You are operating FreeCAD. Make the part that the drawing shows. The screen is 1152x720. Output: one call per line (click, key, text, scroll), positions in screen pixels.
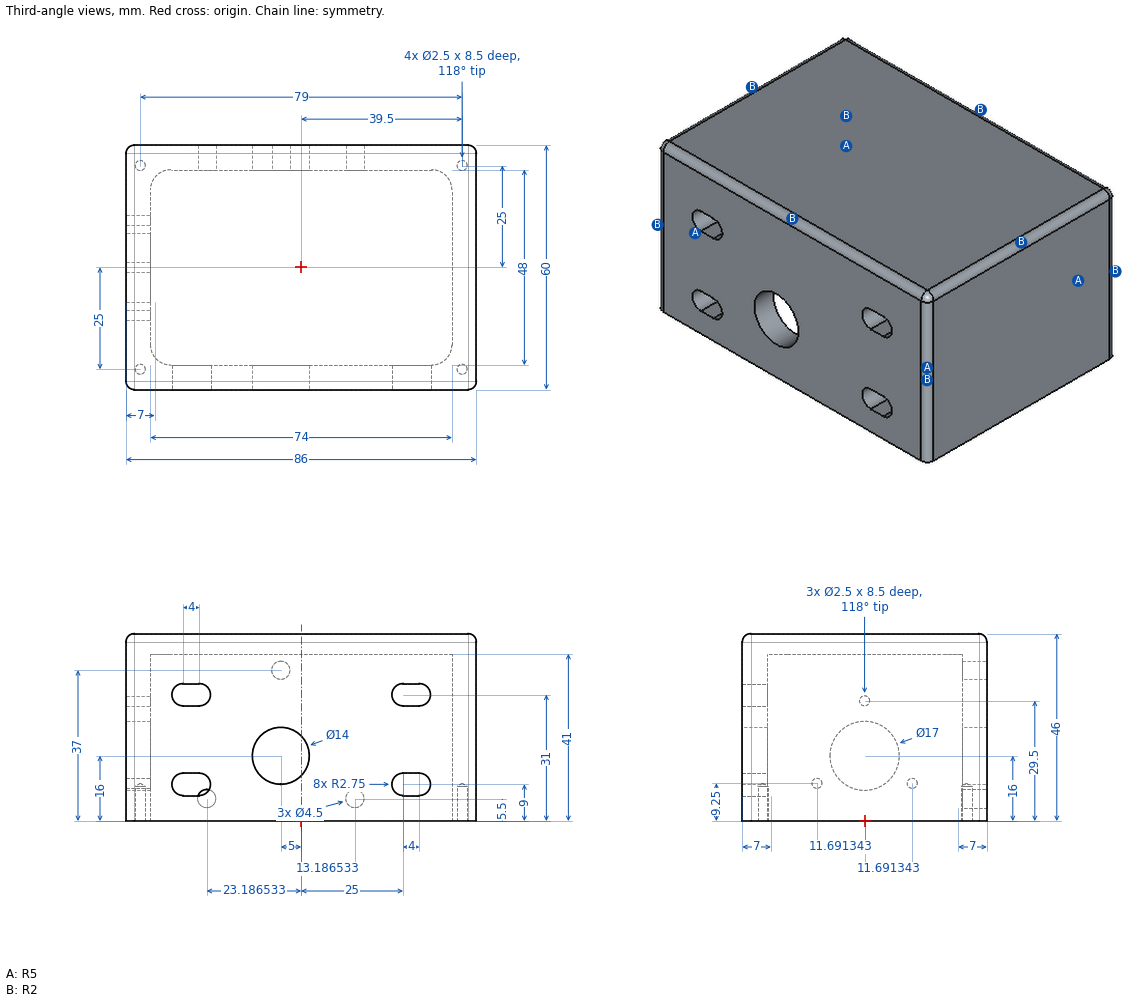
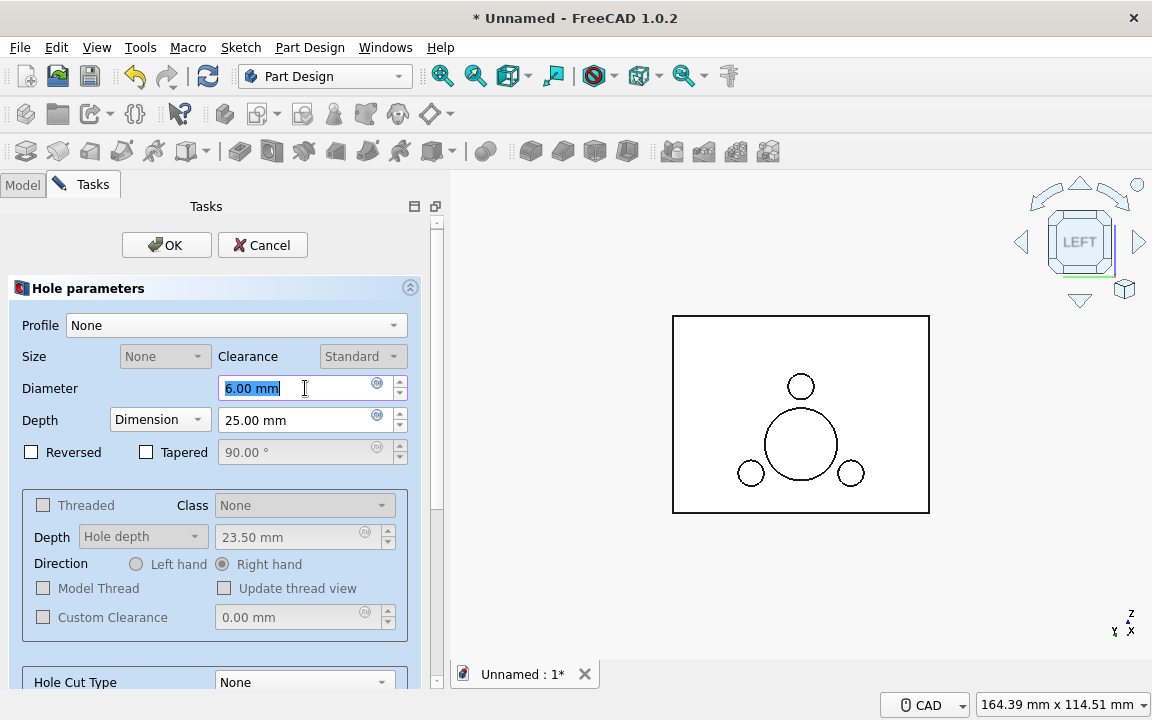
text(2.5)
key(Tab)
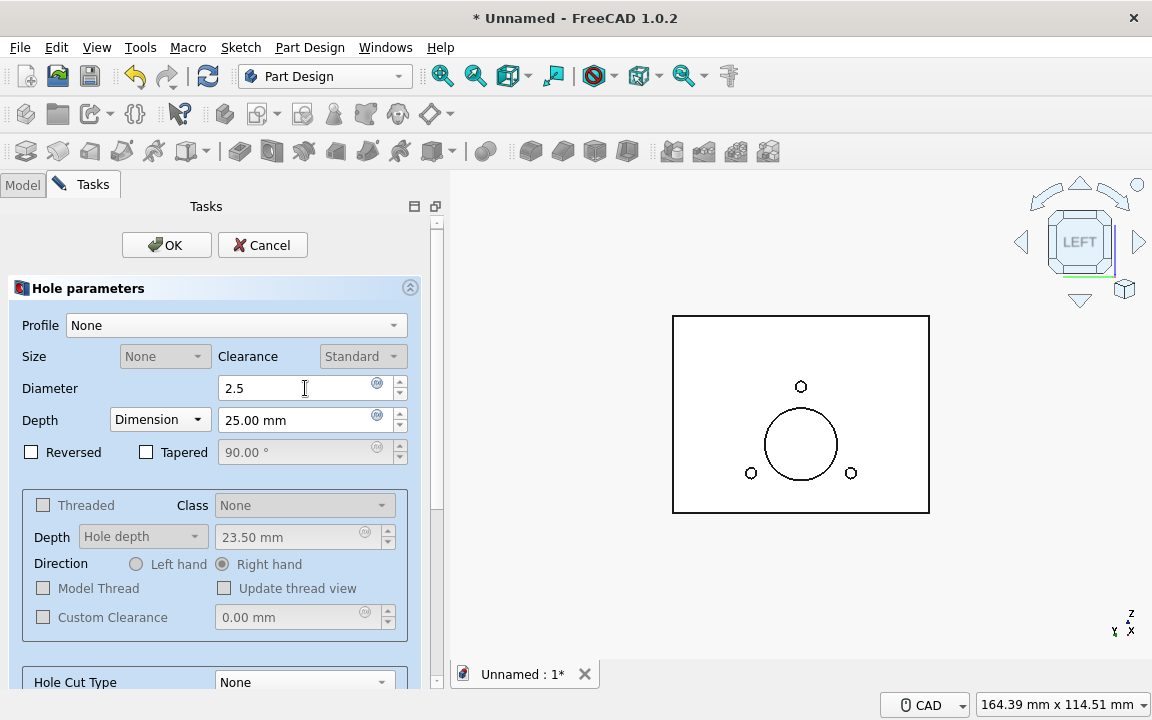
triple_click(305, 420)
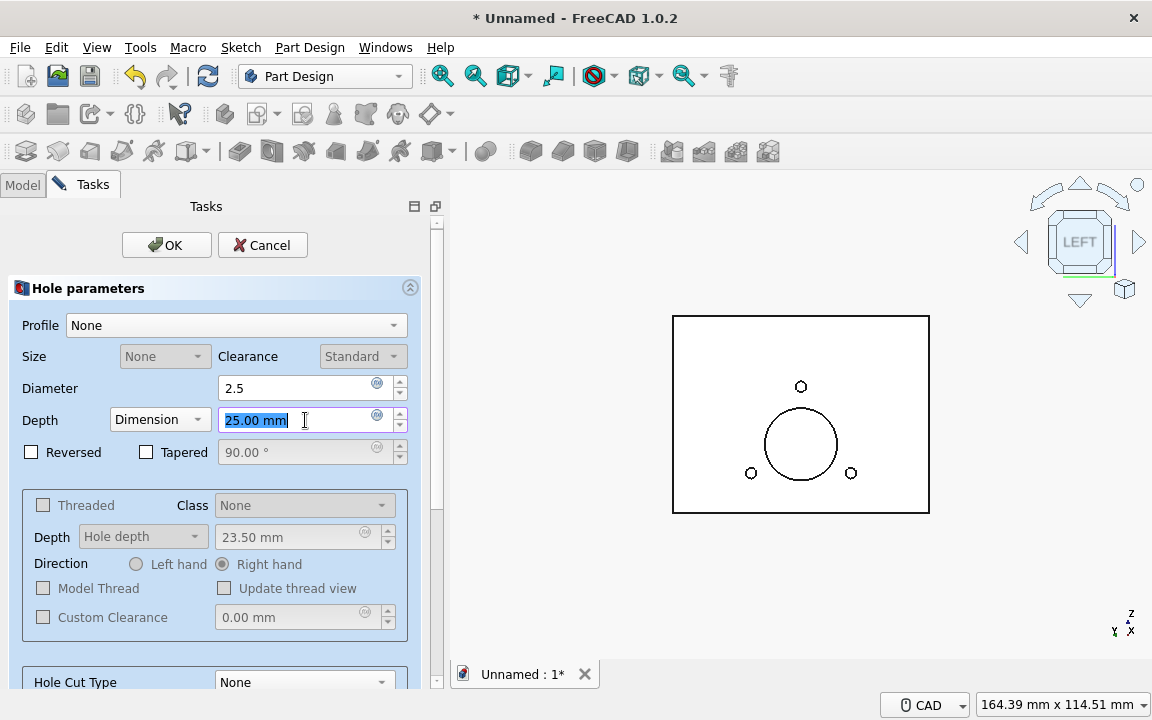
text(8.5)
key(Tab)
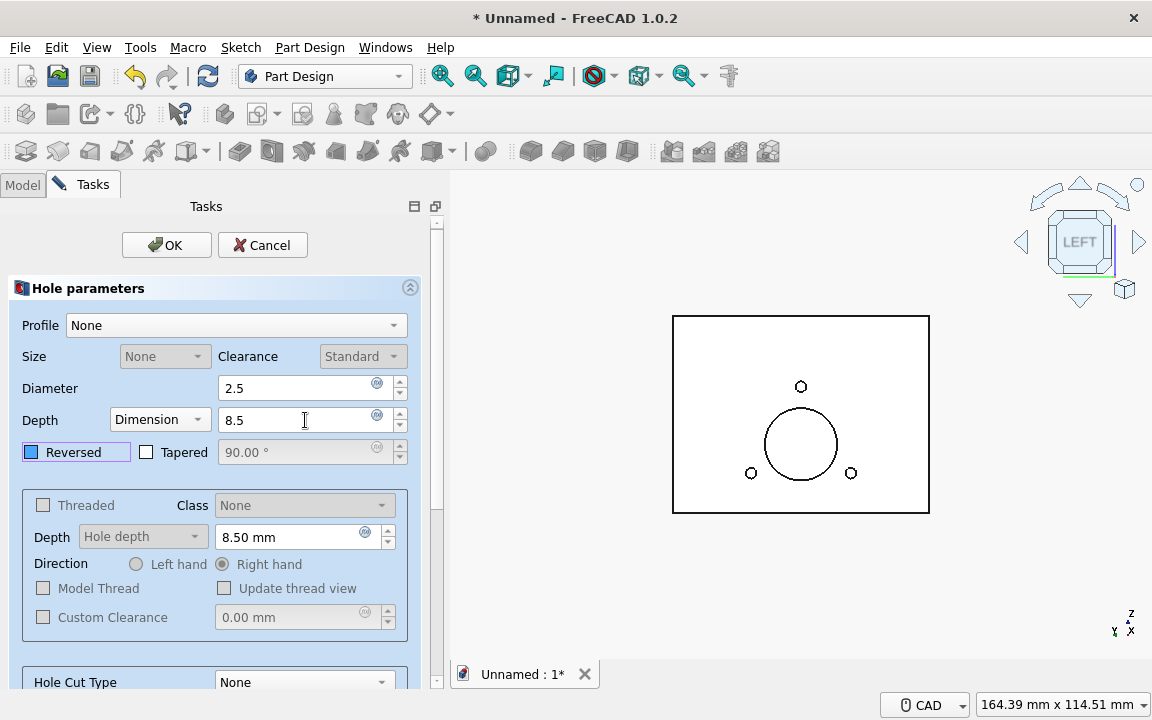
click(167, 245)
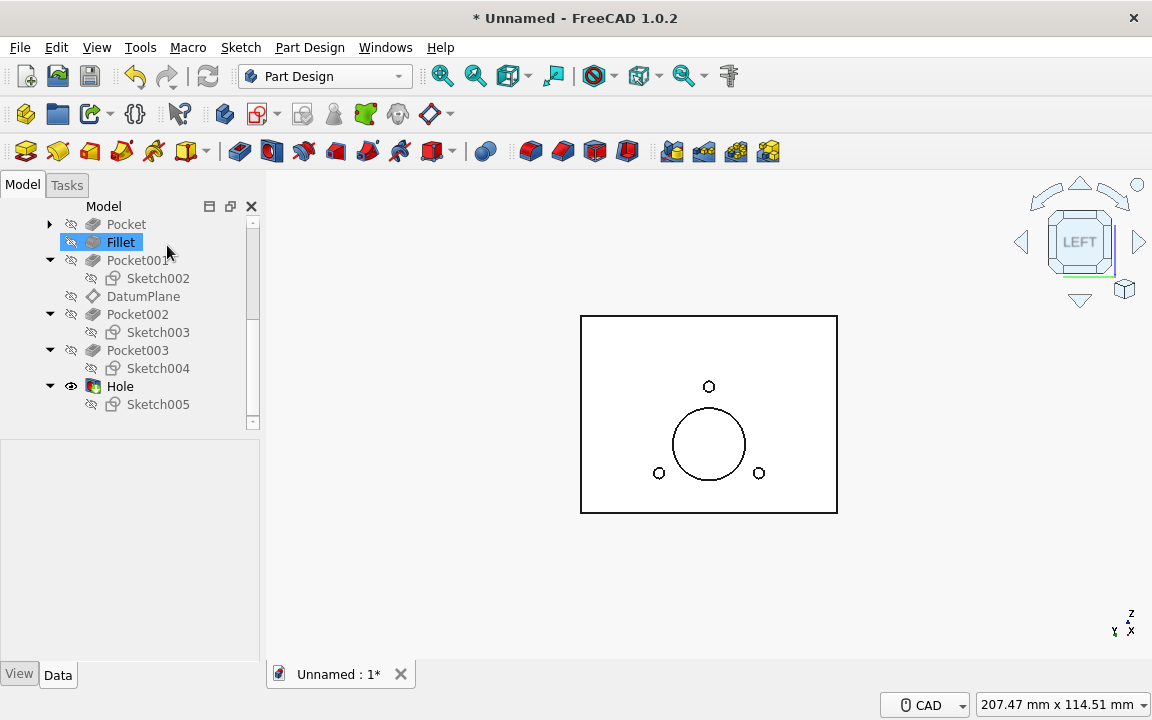
key(v)
key(f)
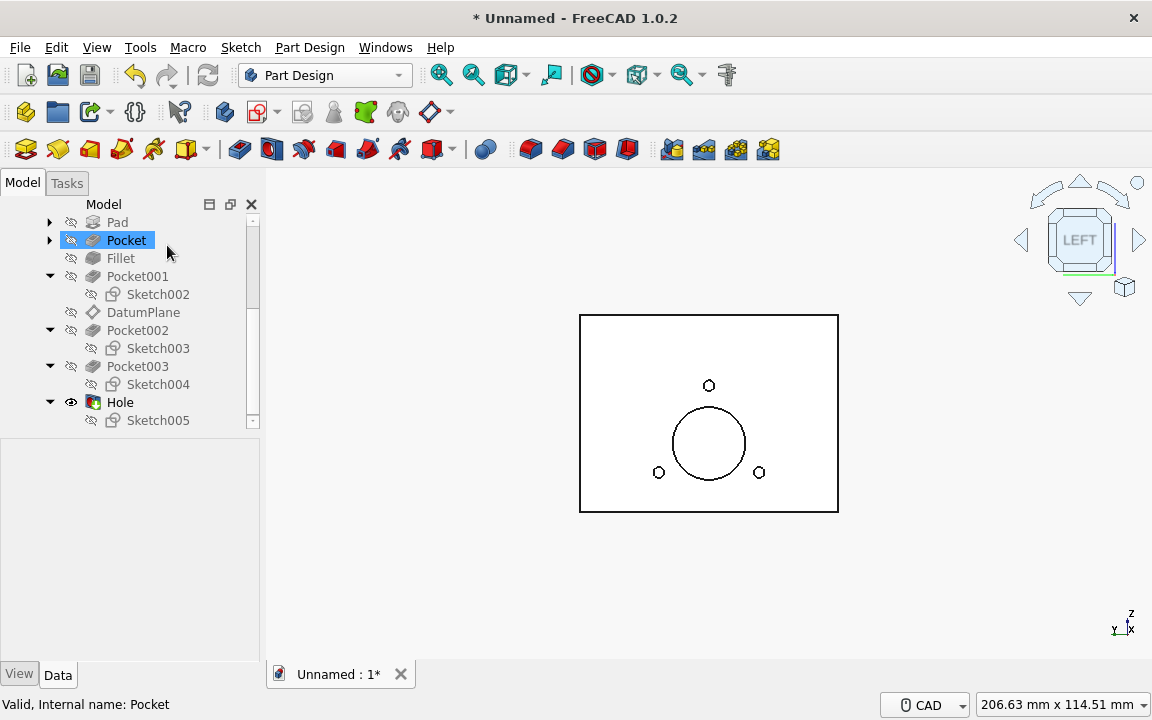
click(258, 112)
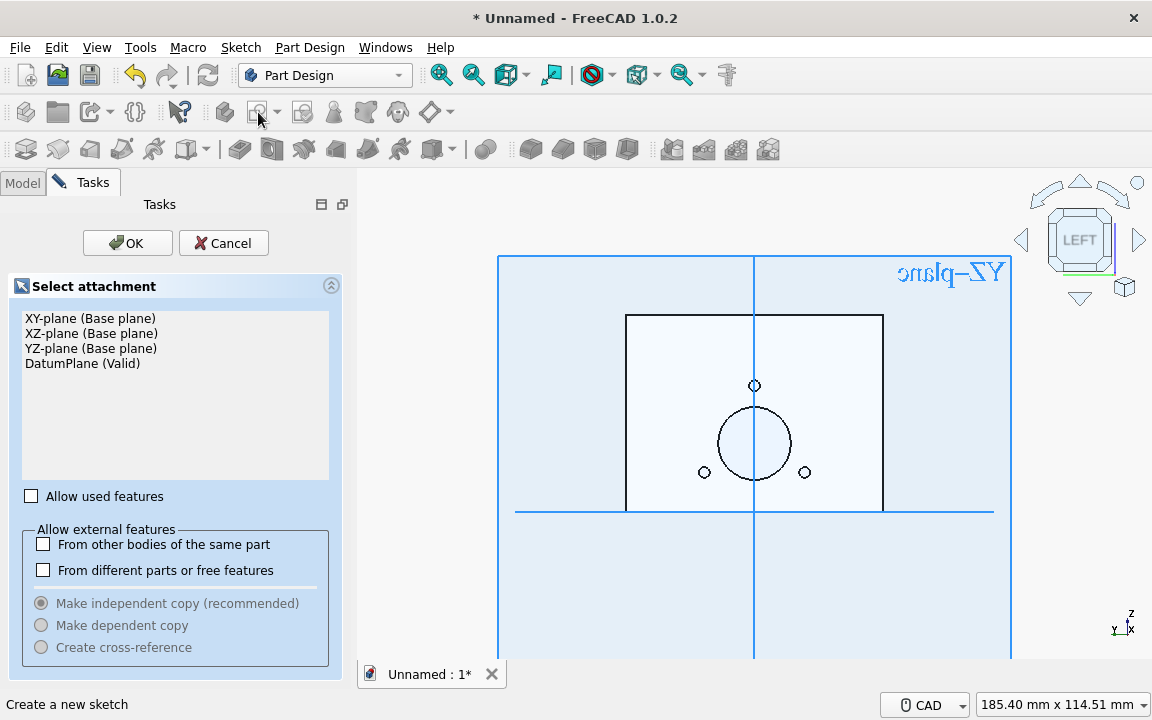
click(82, 318)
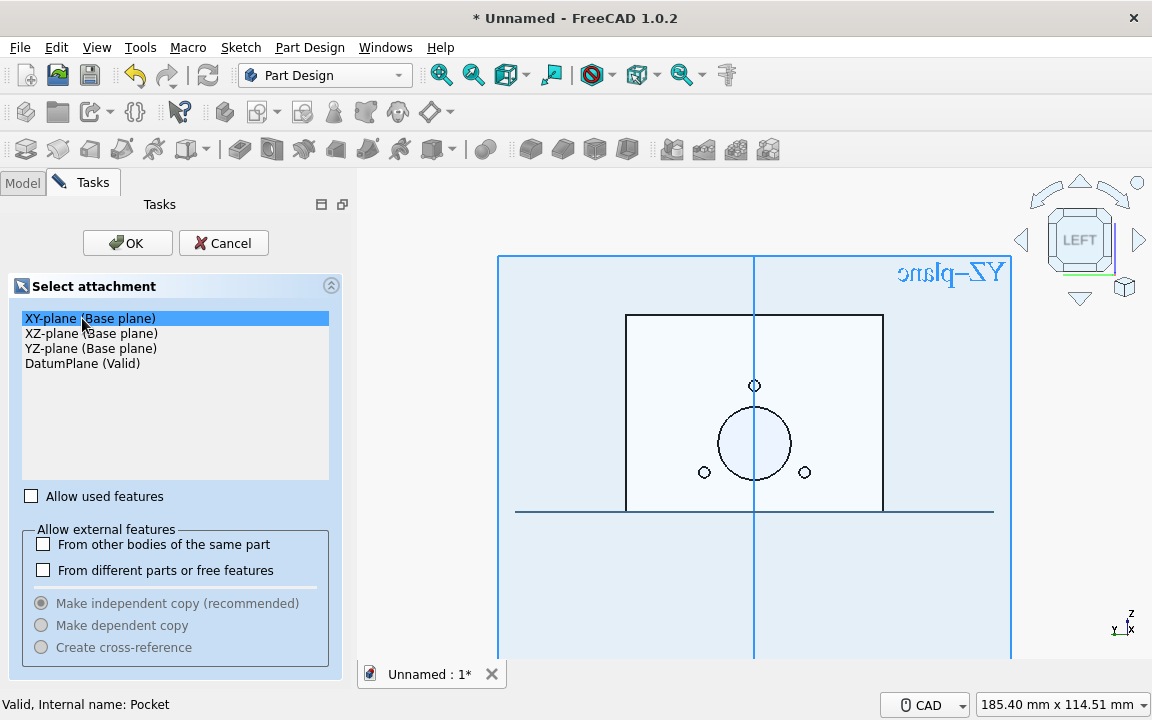
click(128, 243)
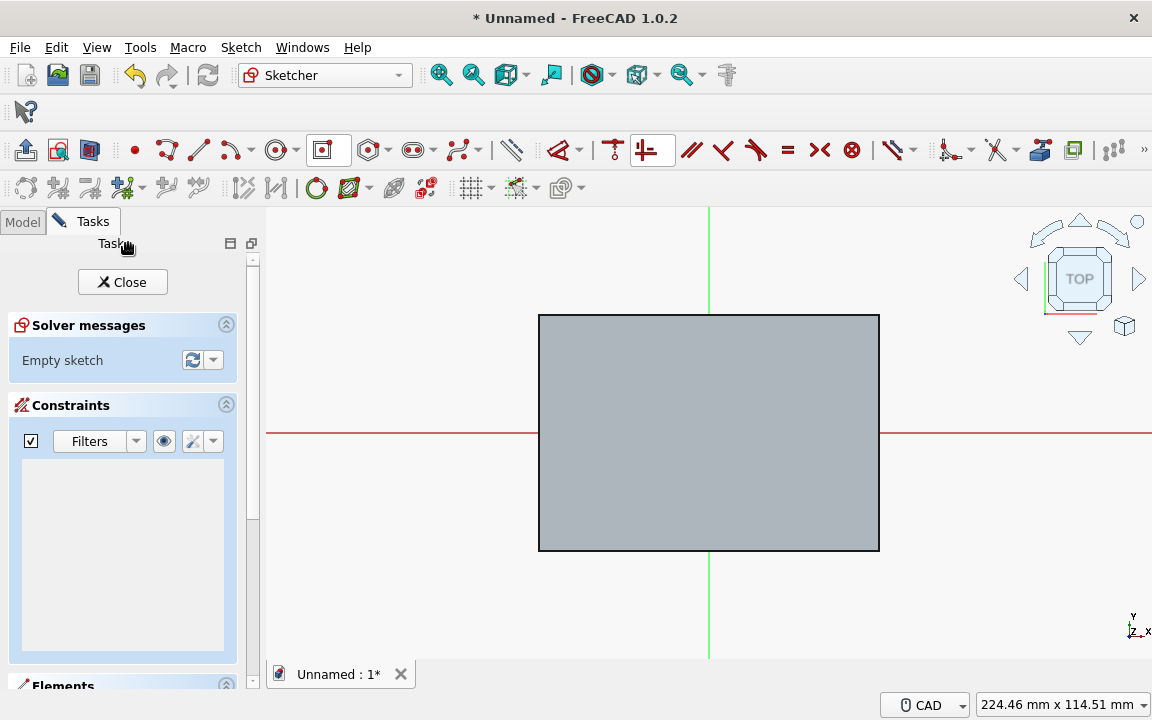
key(q)
key(s)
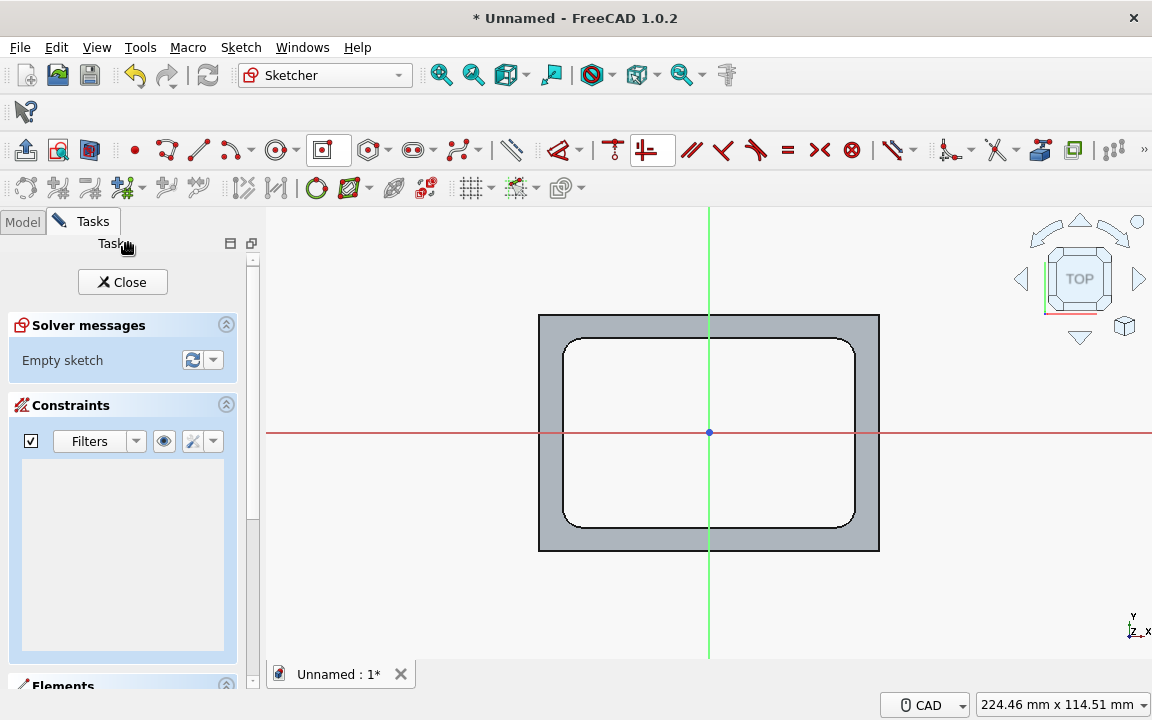
click(276, 150)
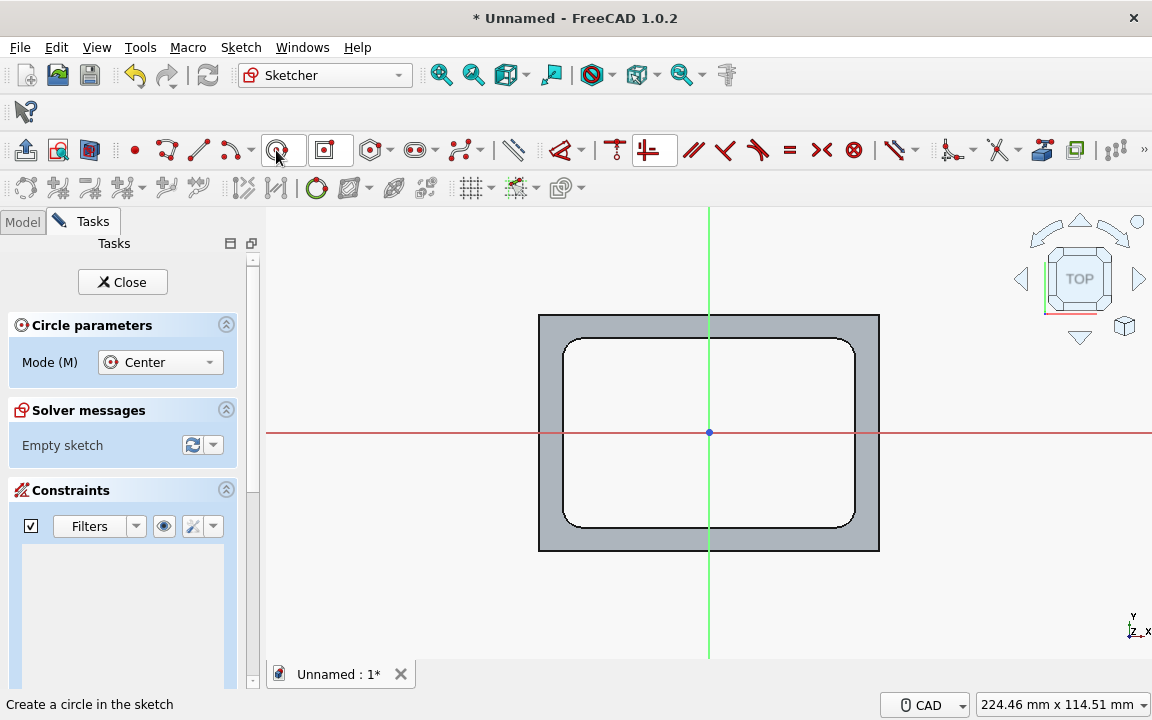
scroll(865, 334, up, 8)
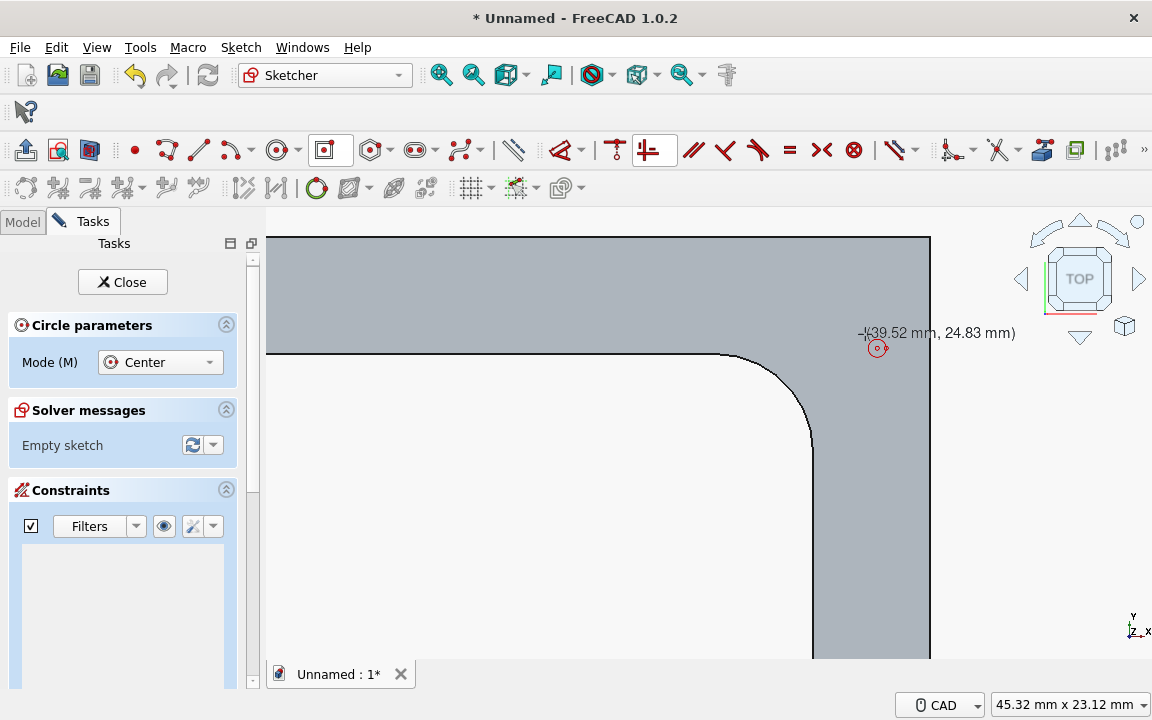
scroll(821, 305, down, 7)